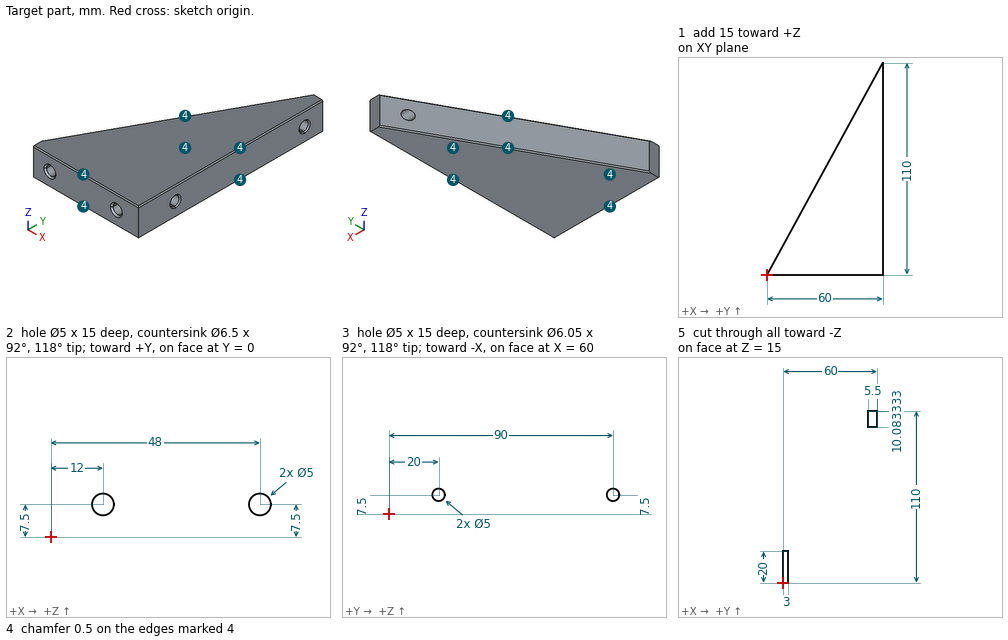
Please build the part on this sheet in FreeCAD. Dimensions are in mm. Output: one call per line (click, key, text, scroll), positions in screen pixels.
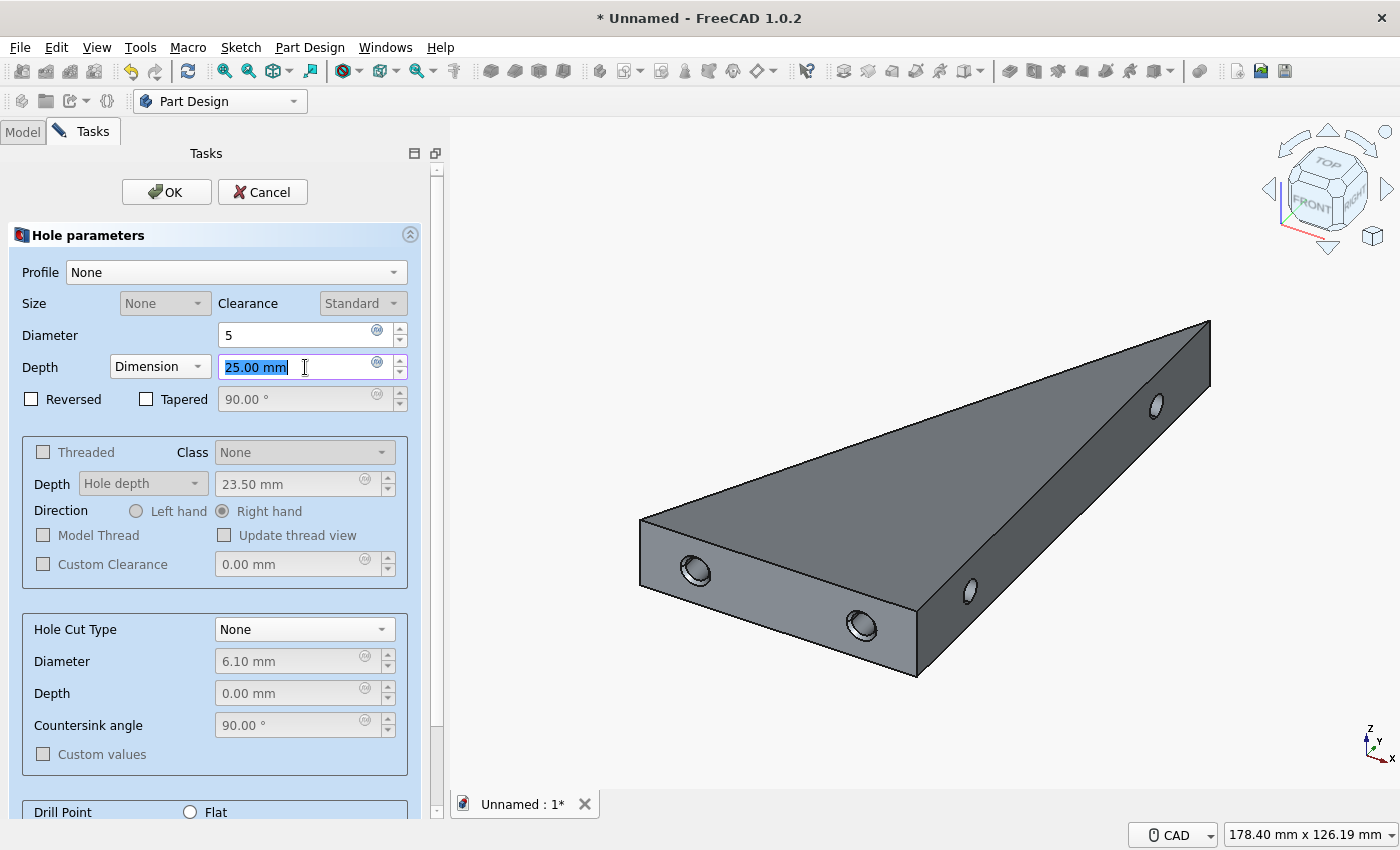
text(15)
key(Tab)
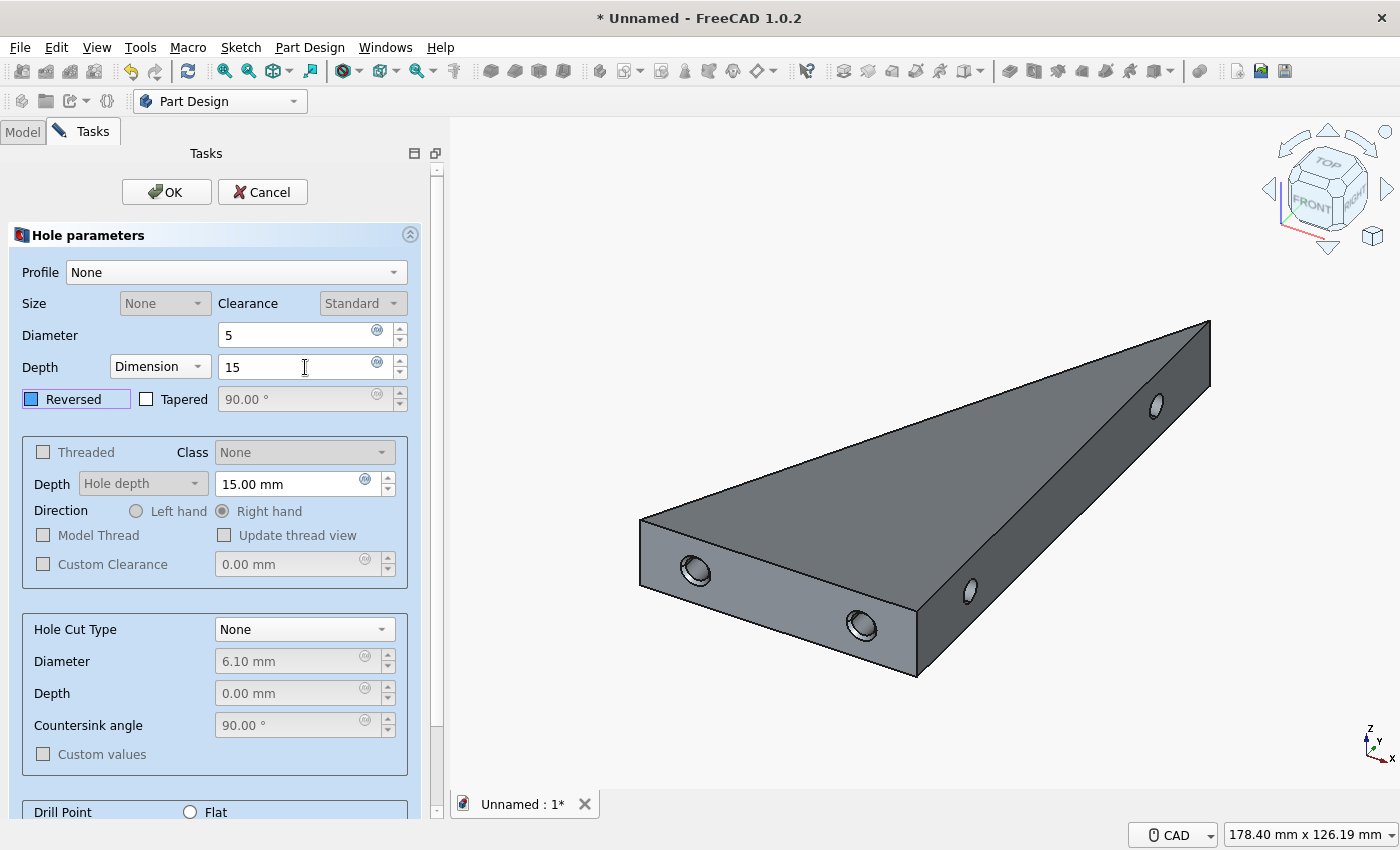
click(306, 630)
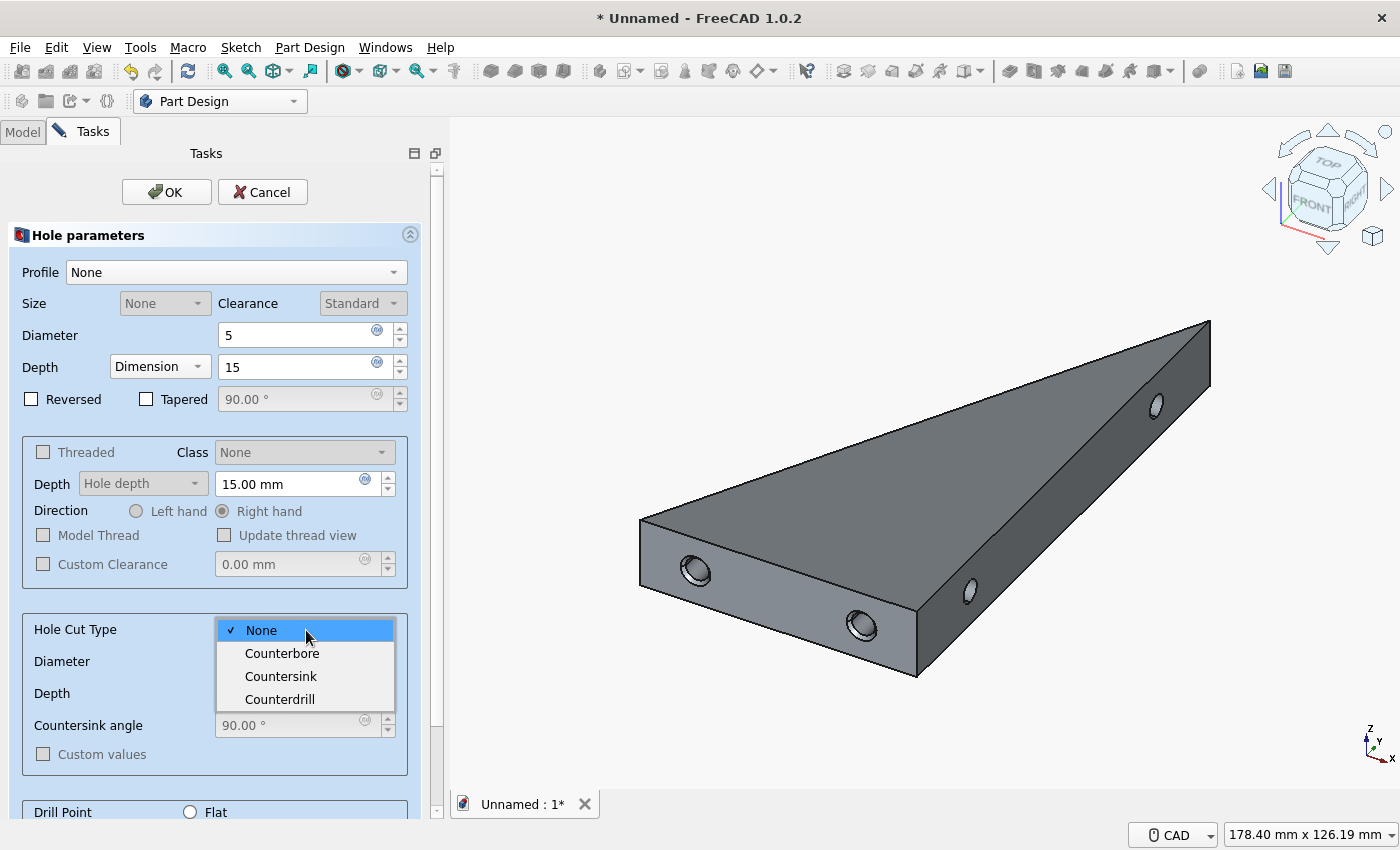
click(304, 676)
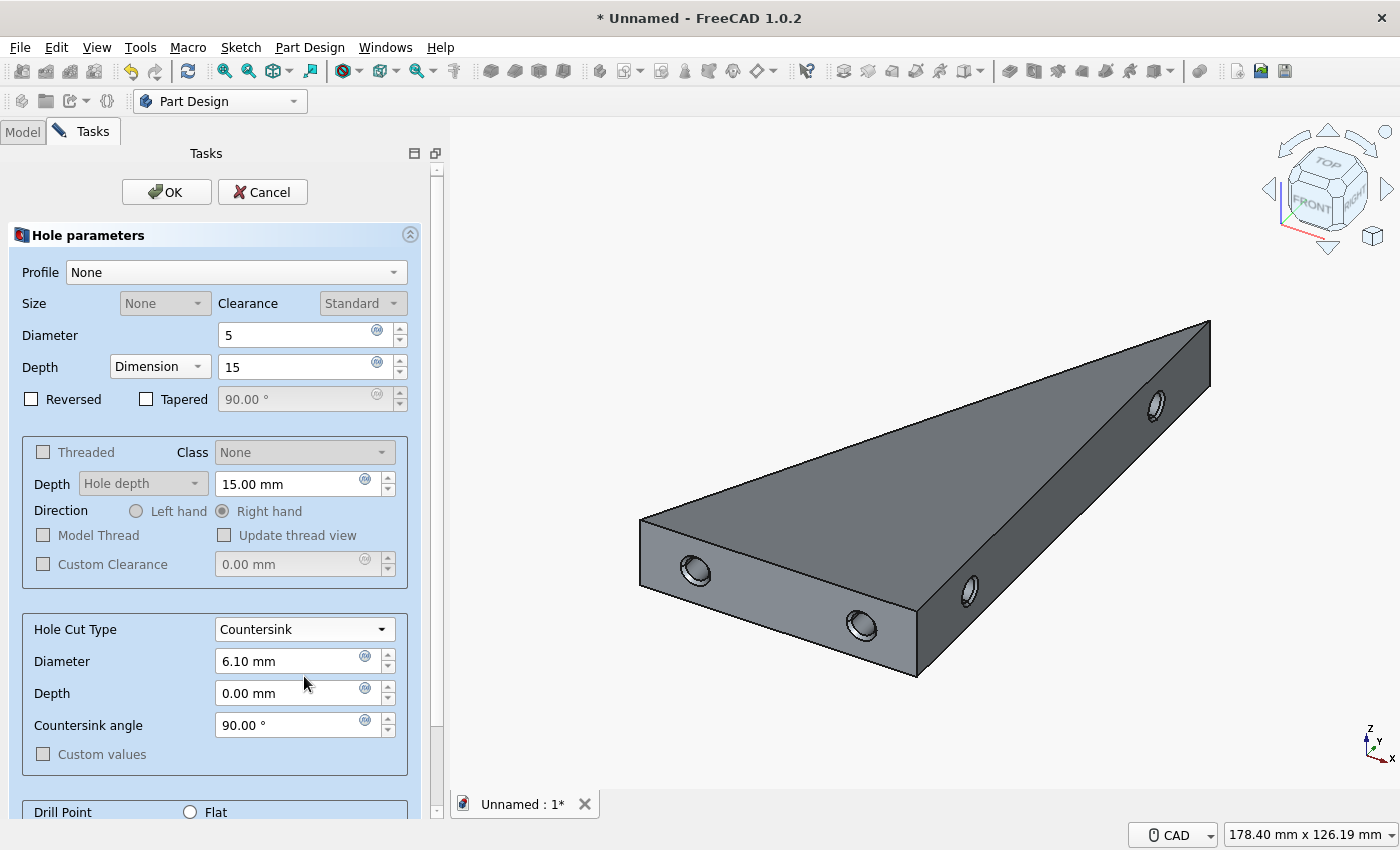
triple_click(298, 725)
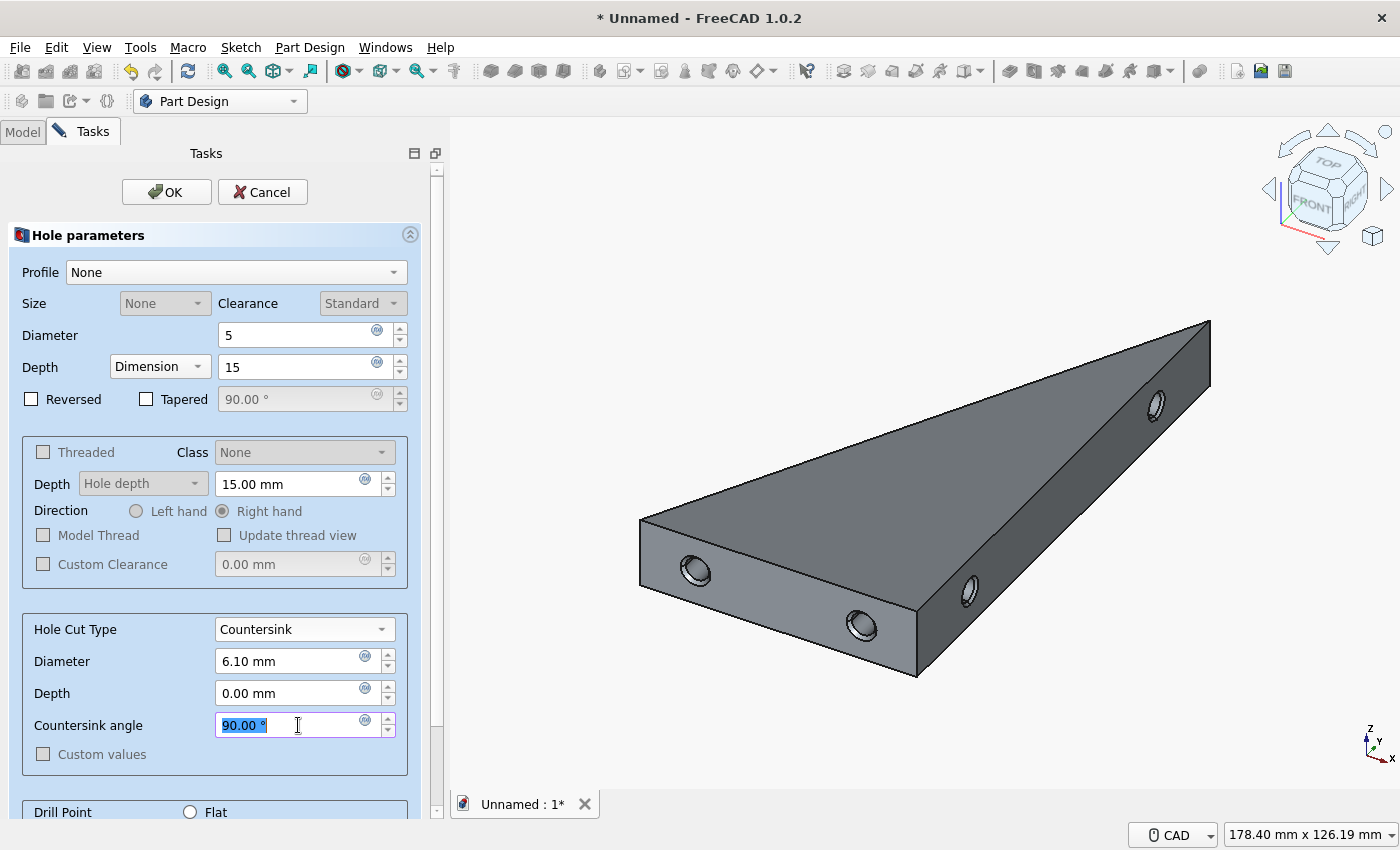
text(92)
key(Tab)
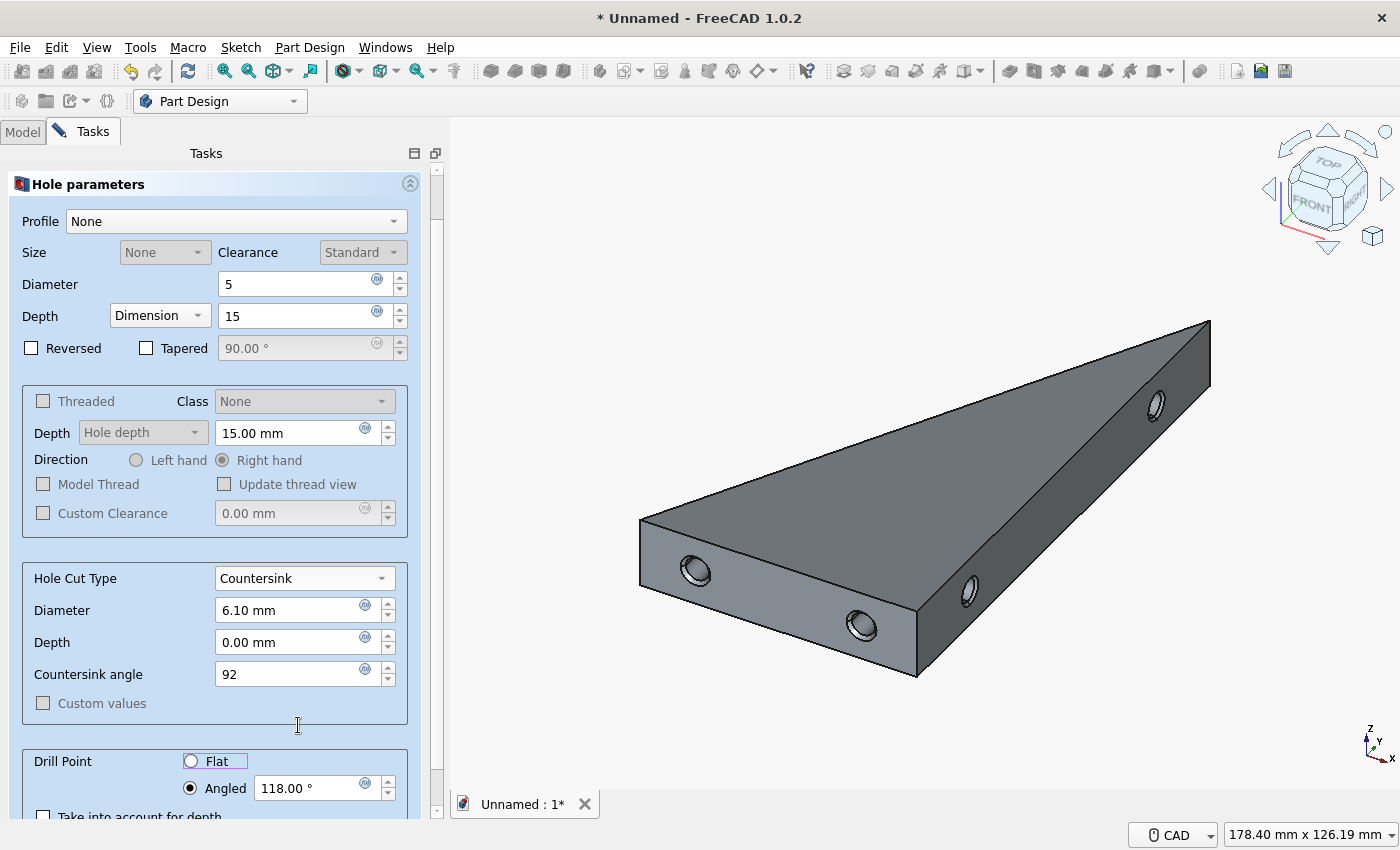
triple_click(298, 610)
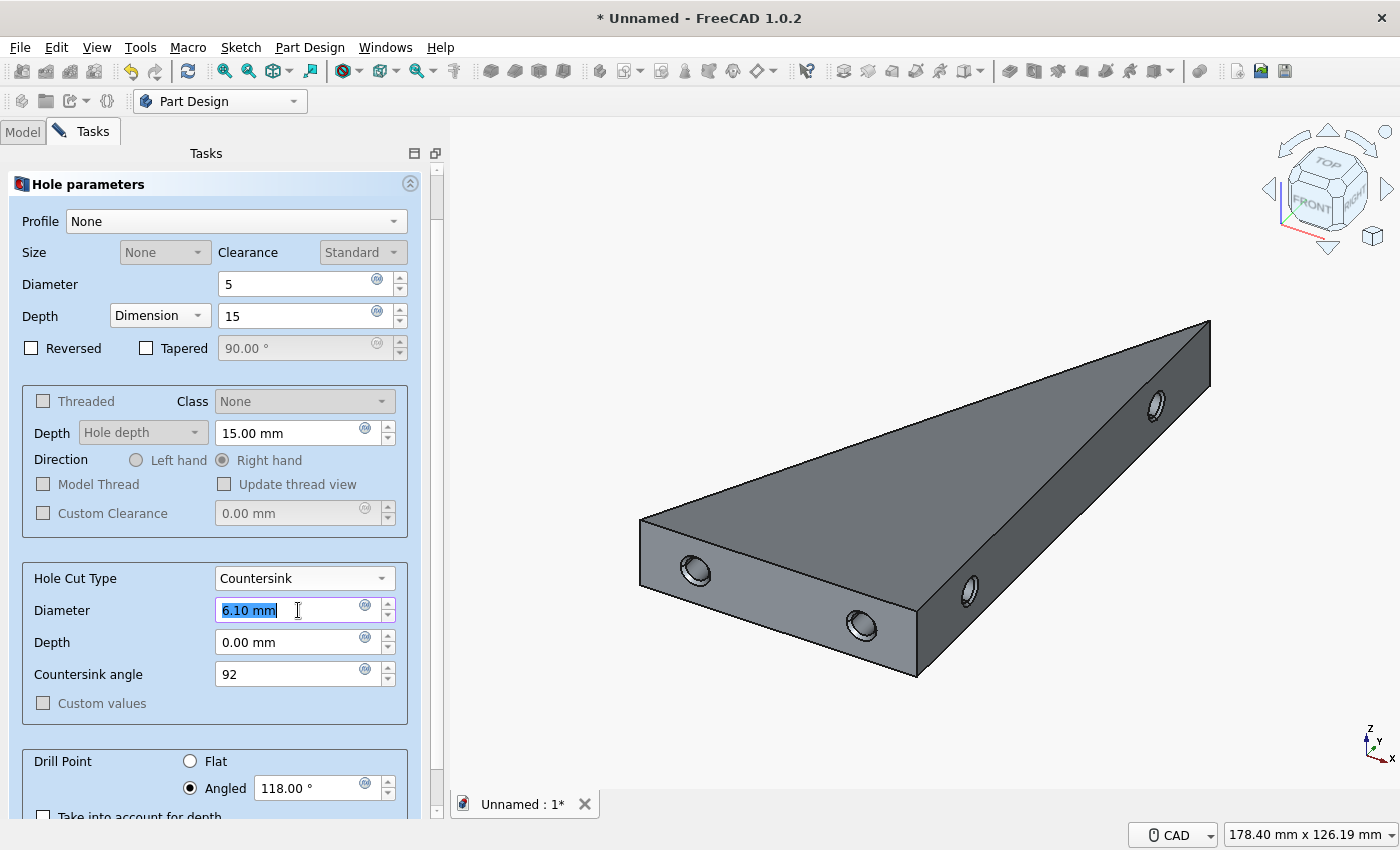
text(6.05)
key(Tab)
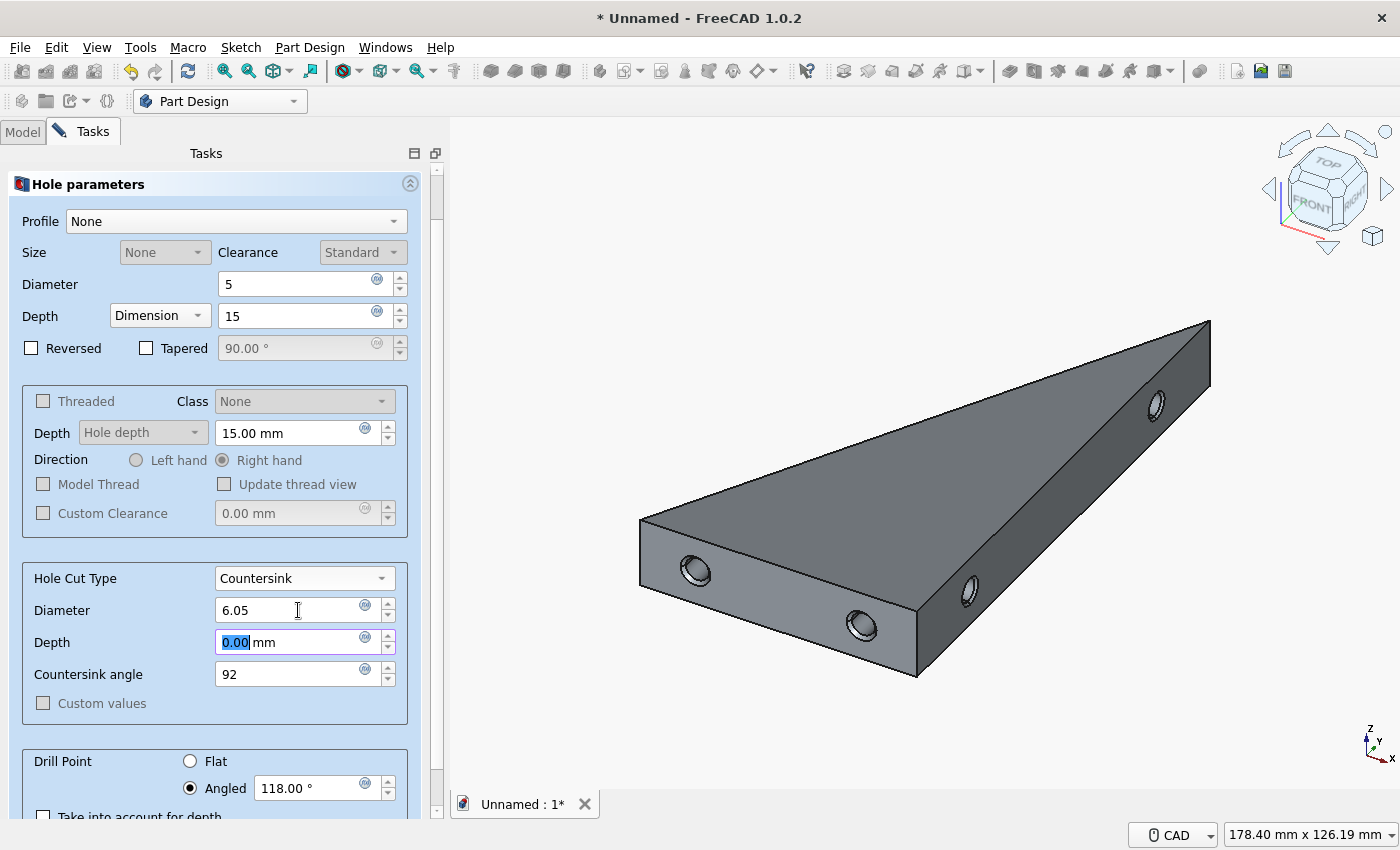
scroll(437, 490, up, 2)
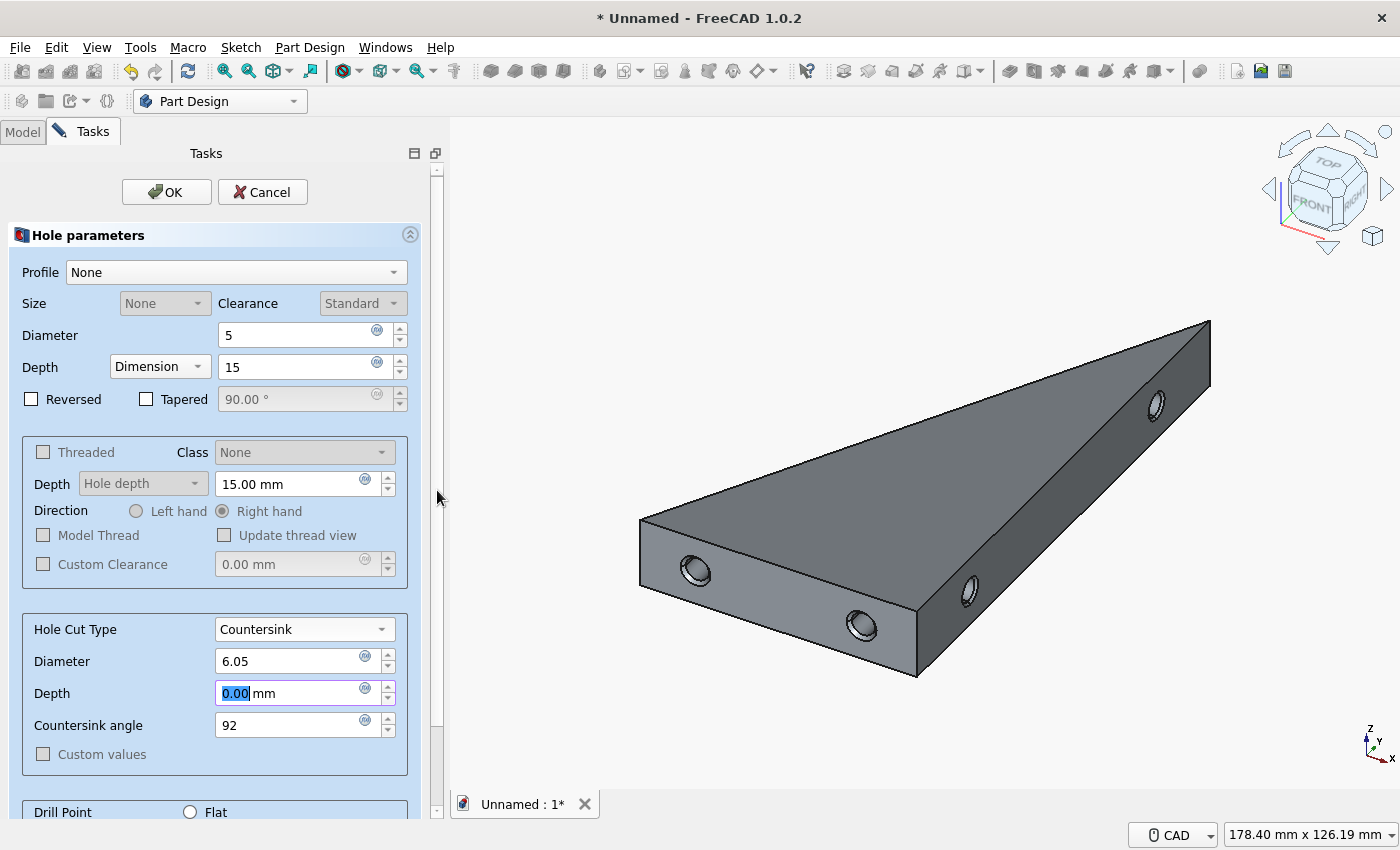
click(167, 192)